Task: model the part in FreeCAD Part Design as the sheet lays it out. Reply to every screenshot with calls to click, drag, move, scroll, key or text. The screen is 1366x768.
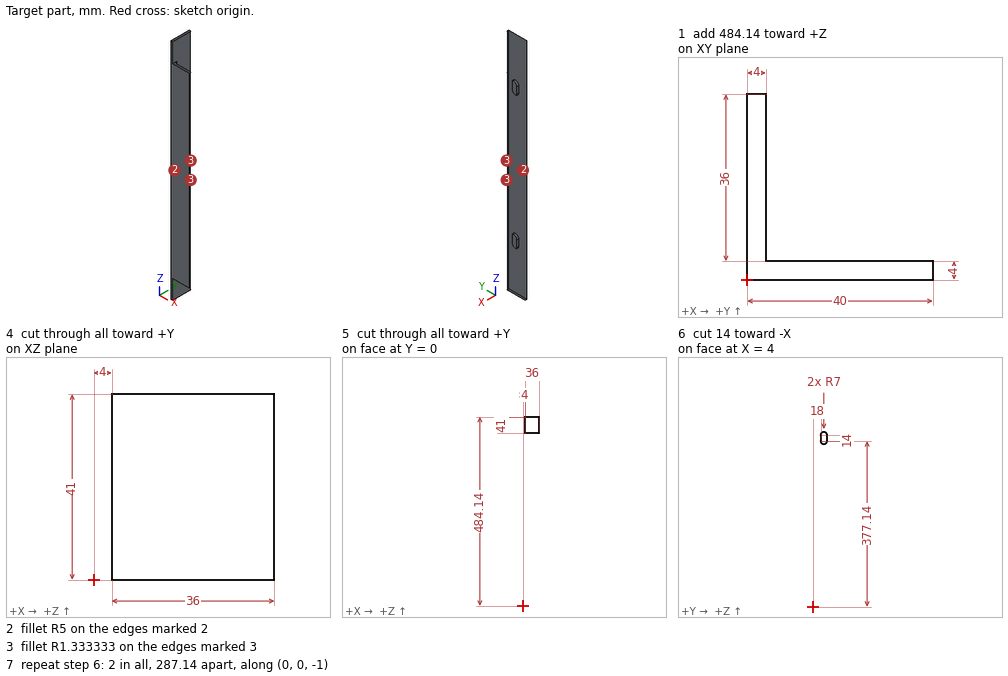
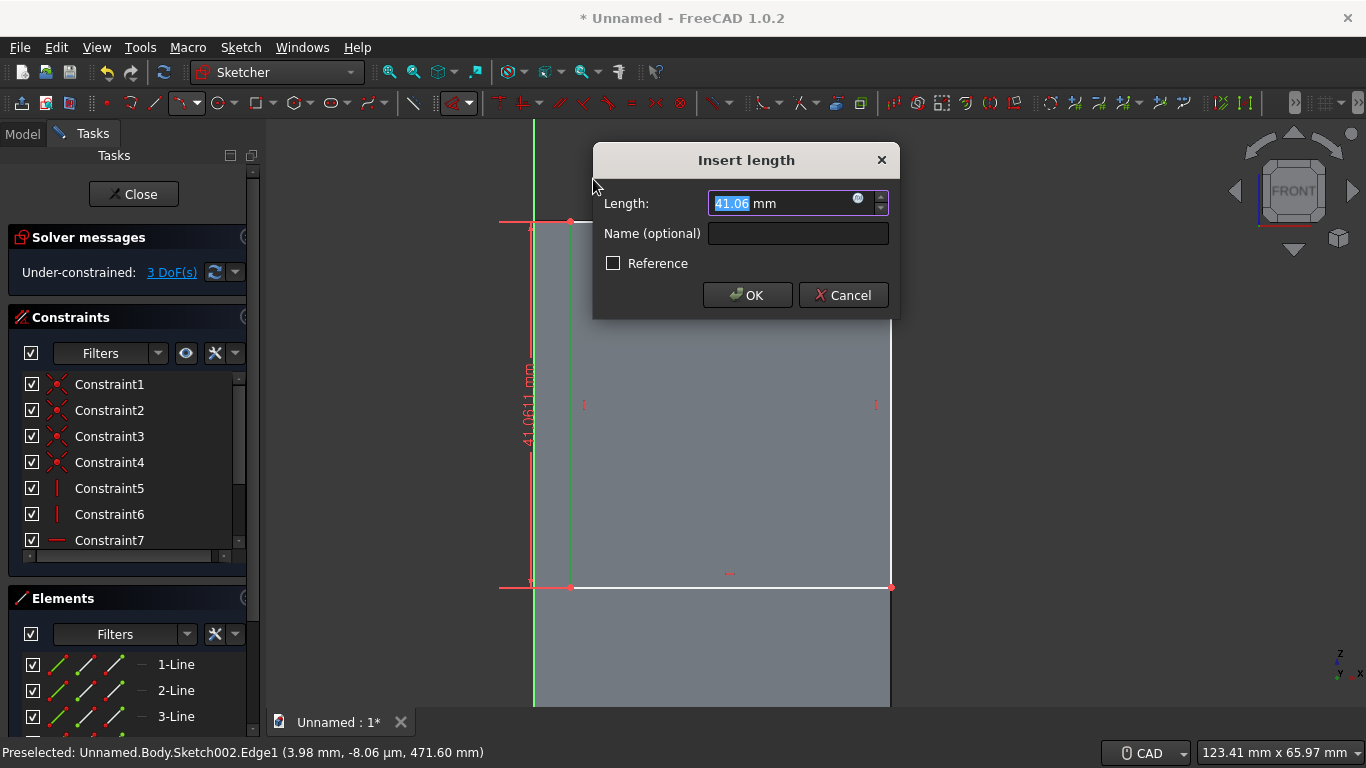
text(41)
key(Return)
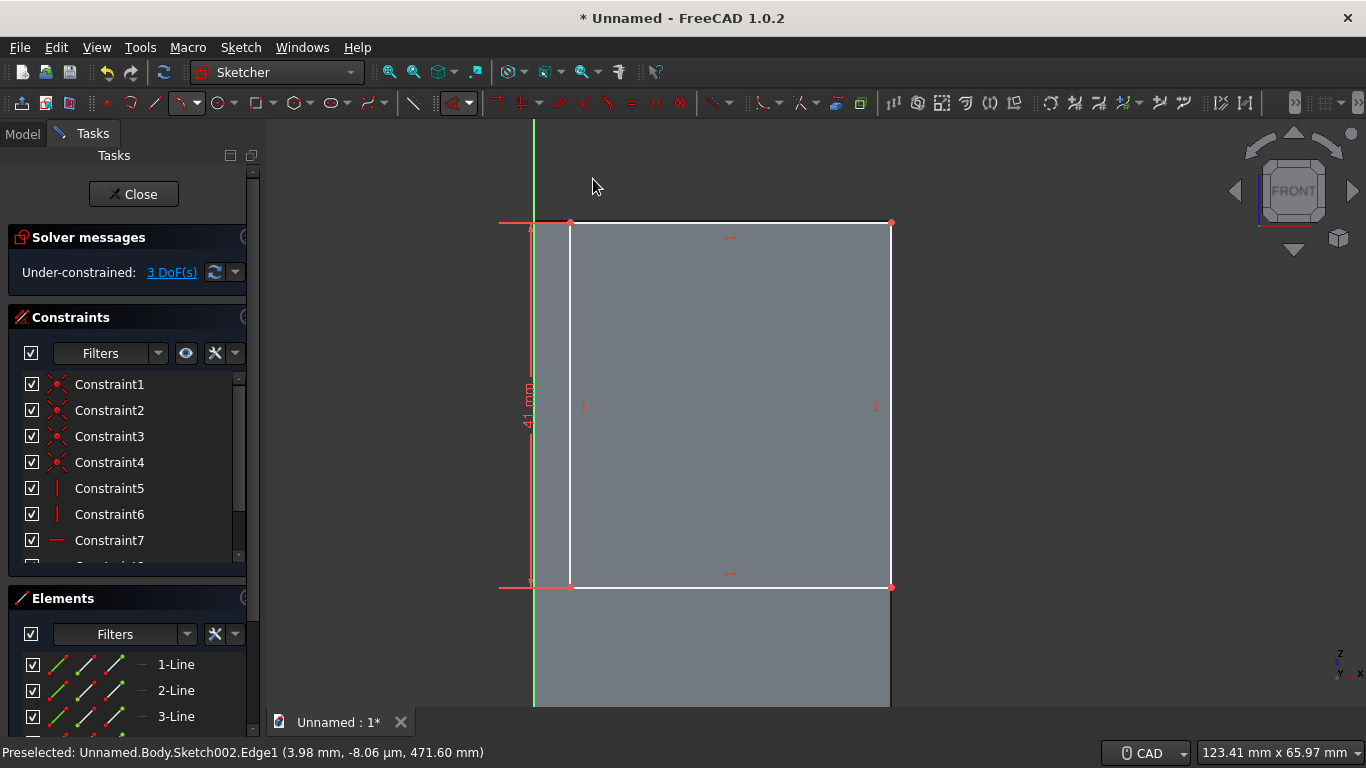
click(666, 588)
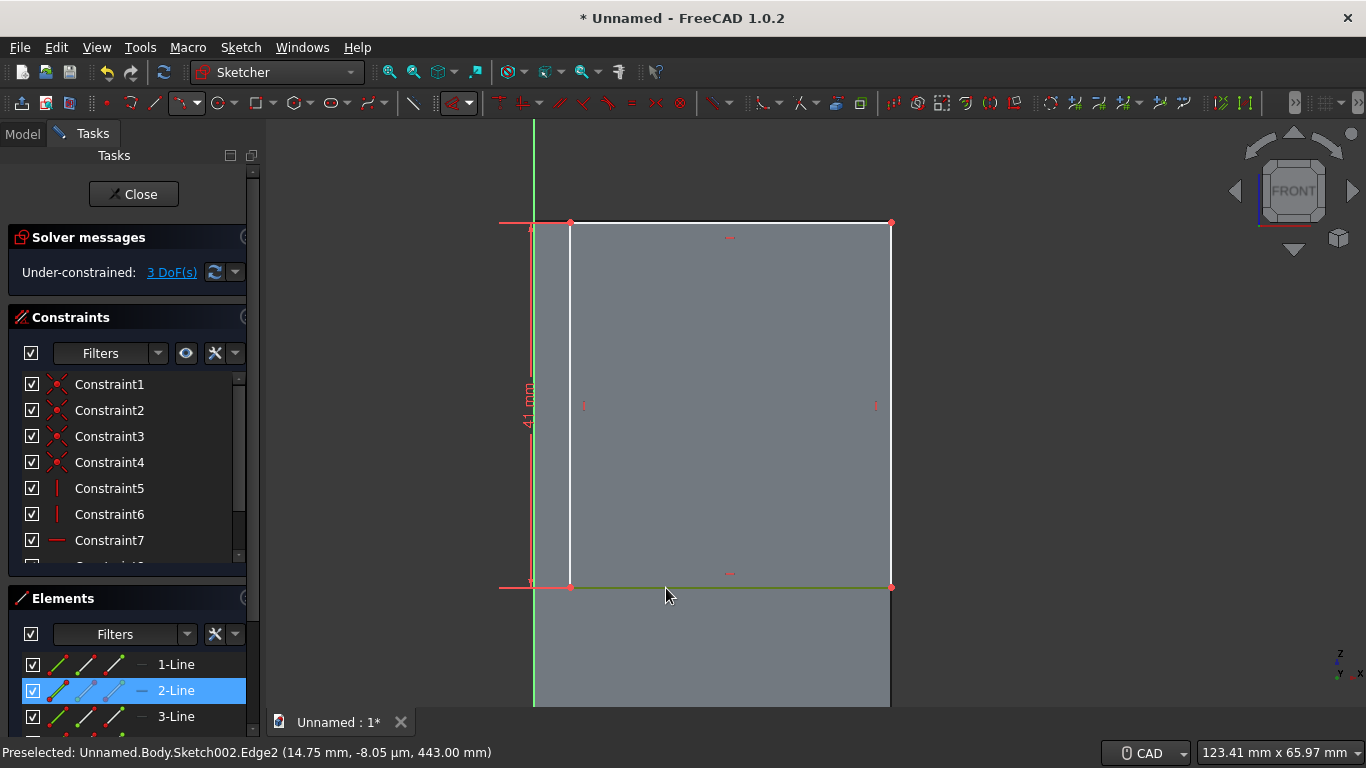
click(472, 104)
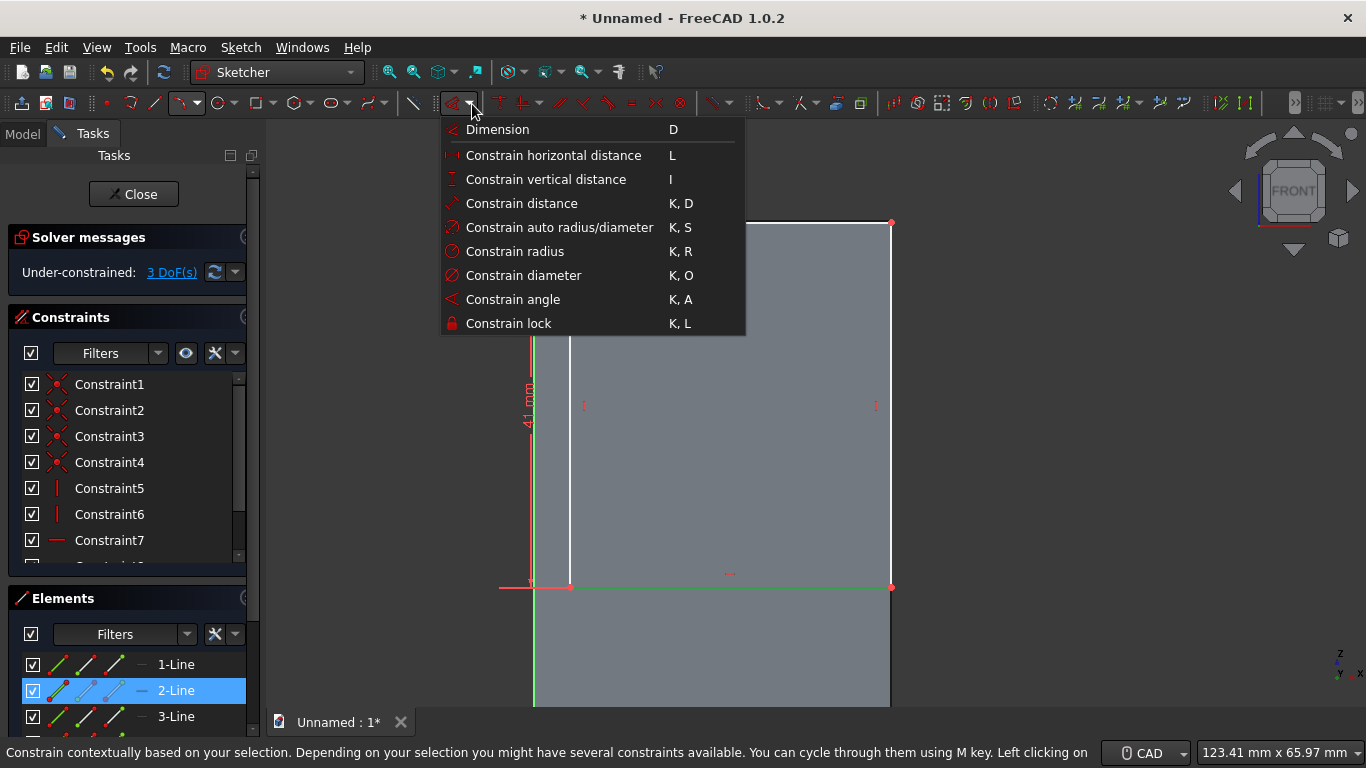
click(593, 155)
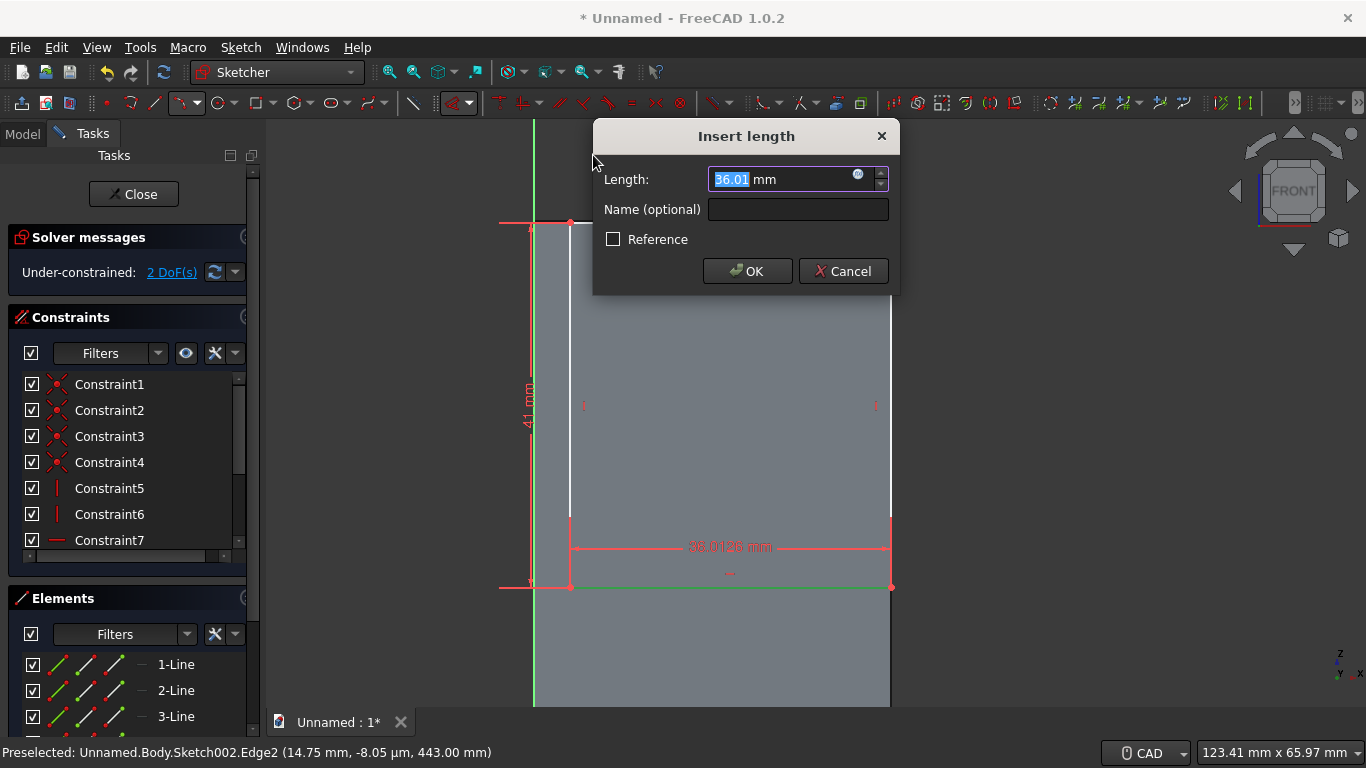
text(36)
key(Return)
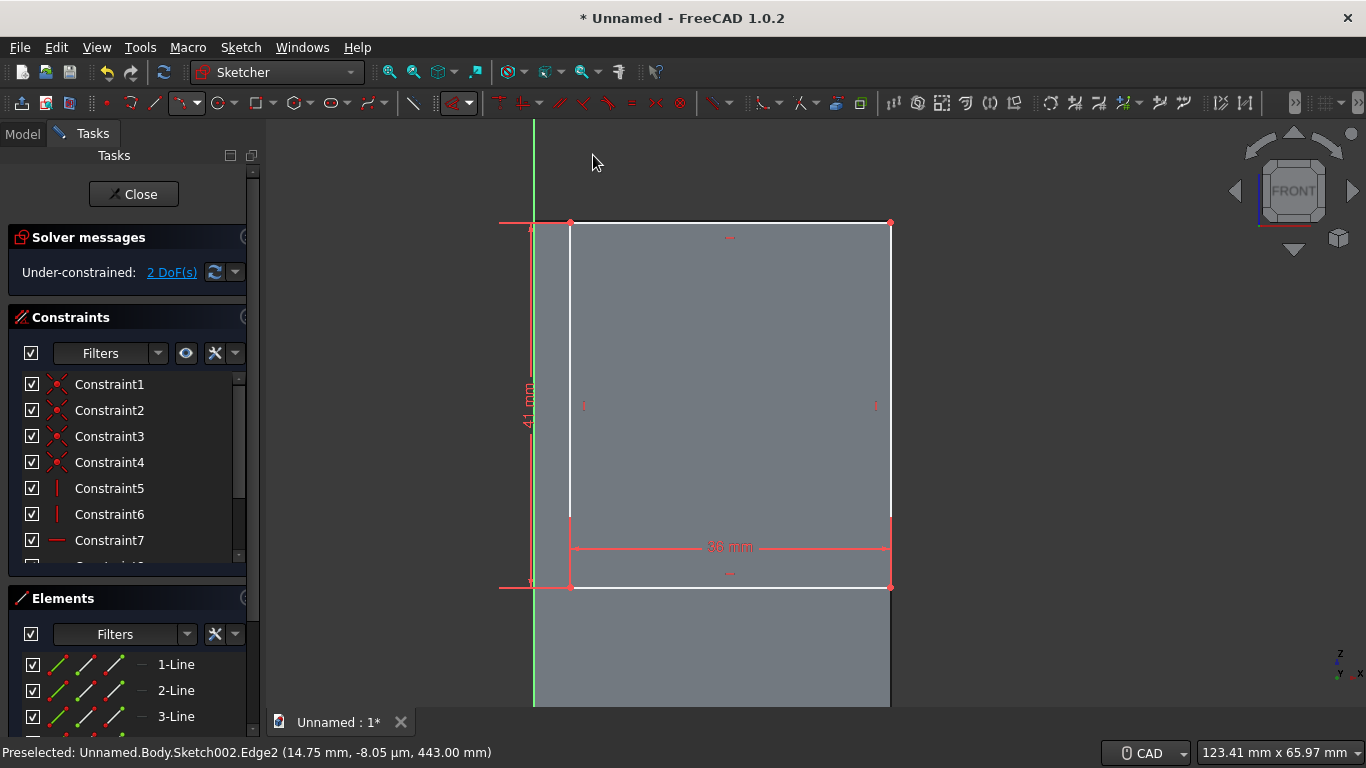
click(570, 223)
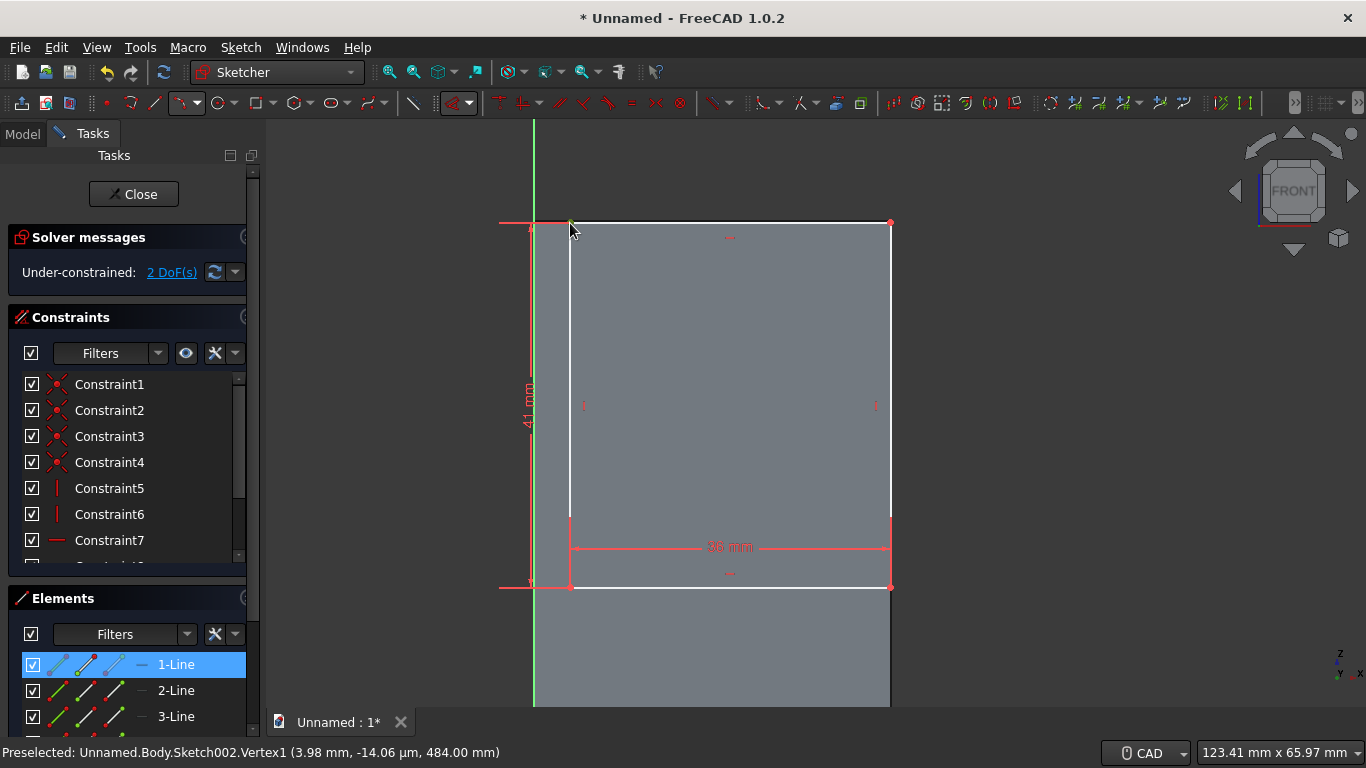
key(l)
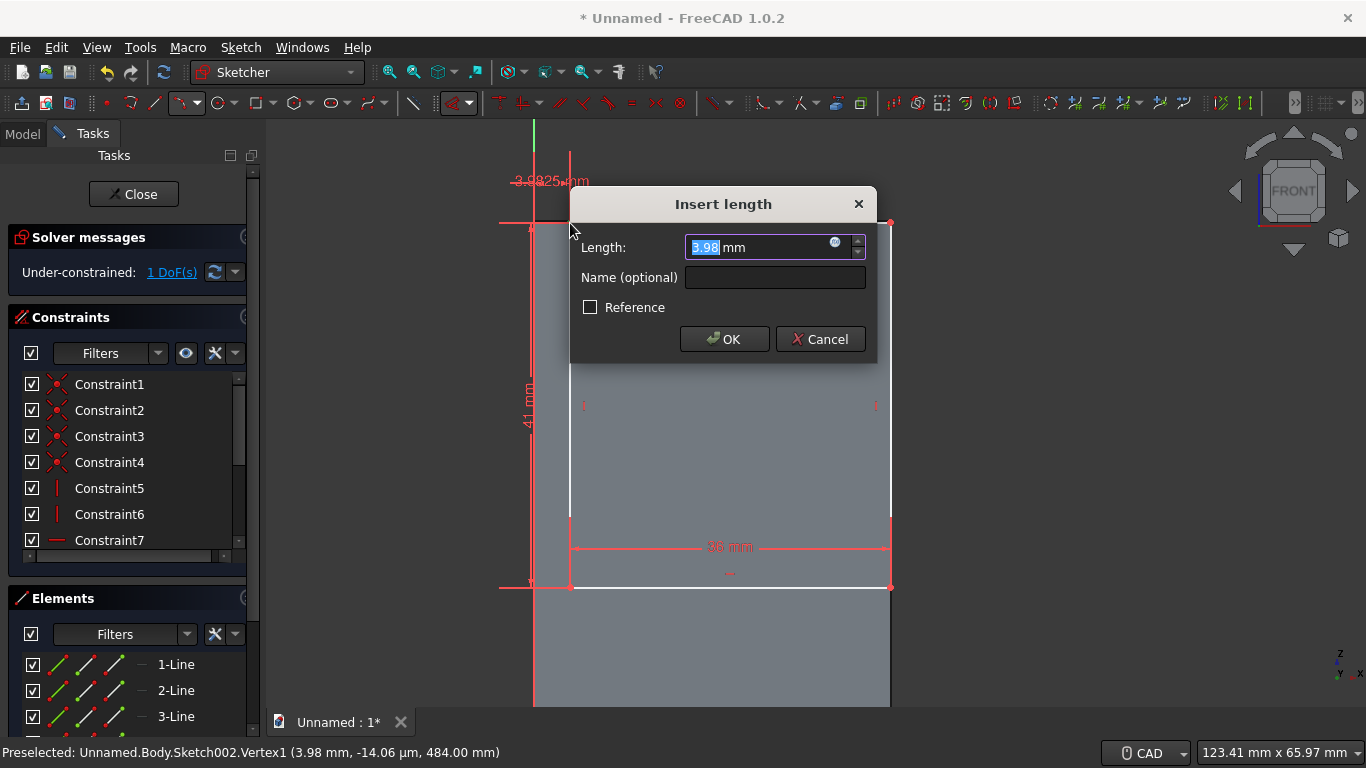
text(4)
key(Return)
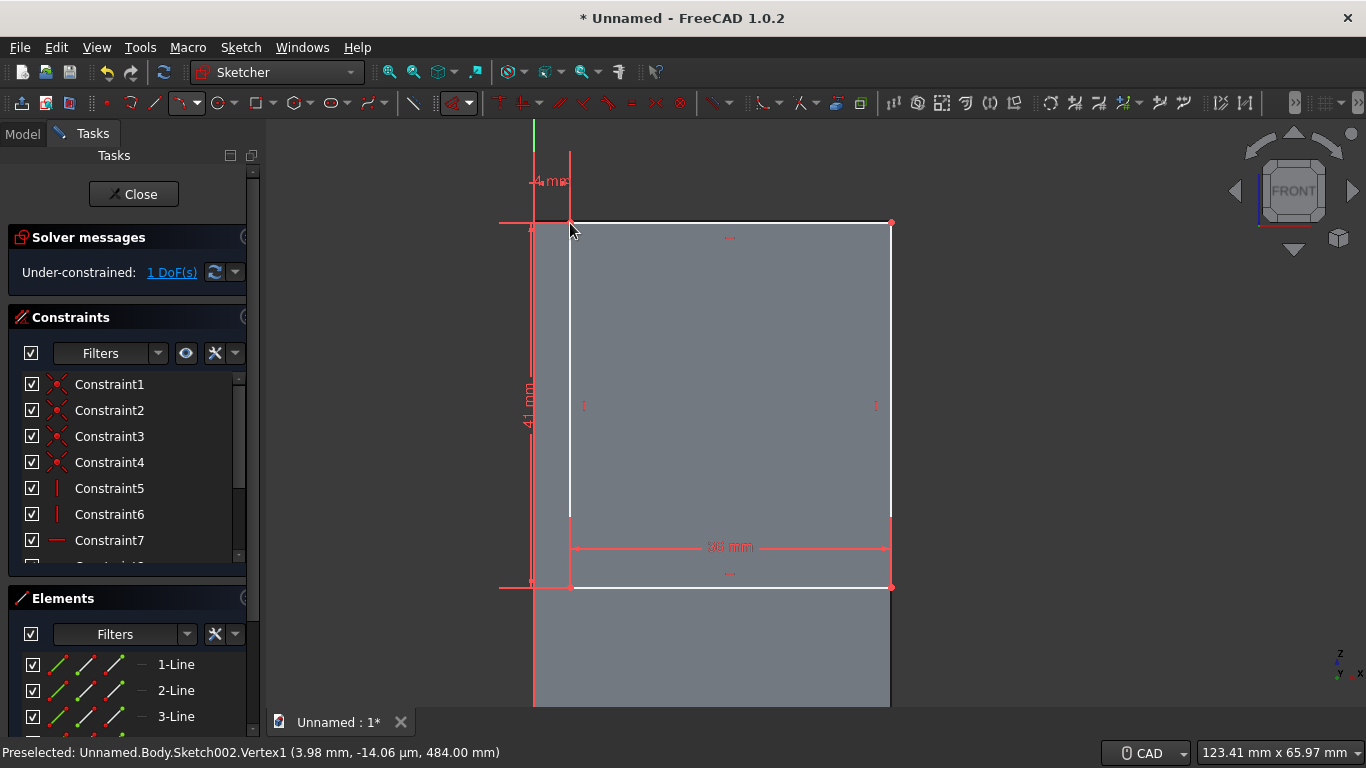
click(570, 223)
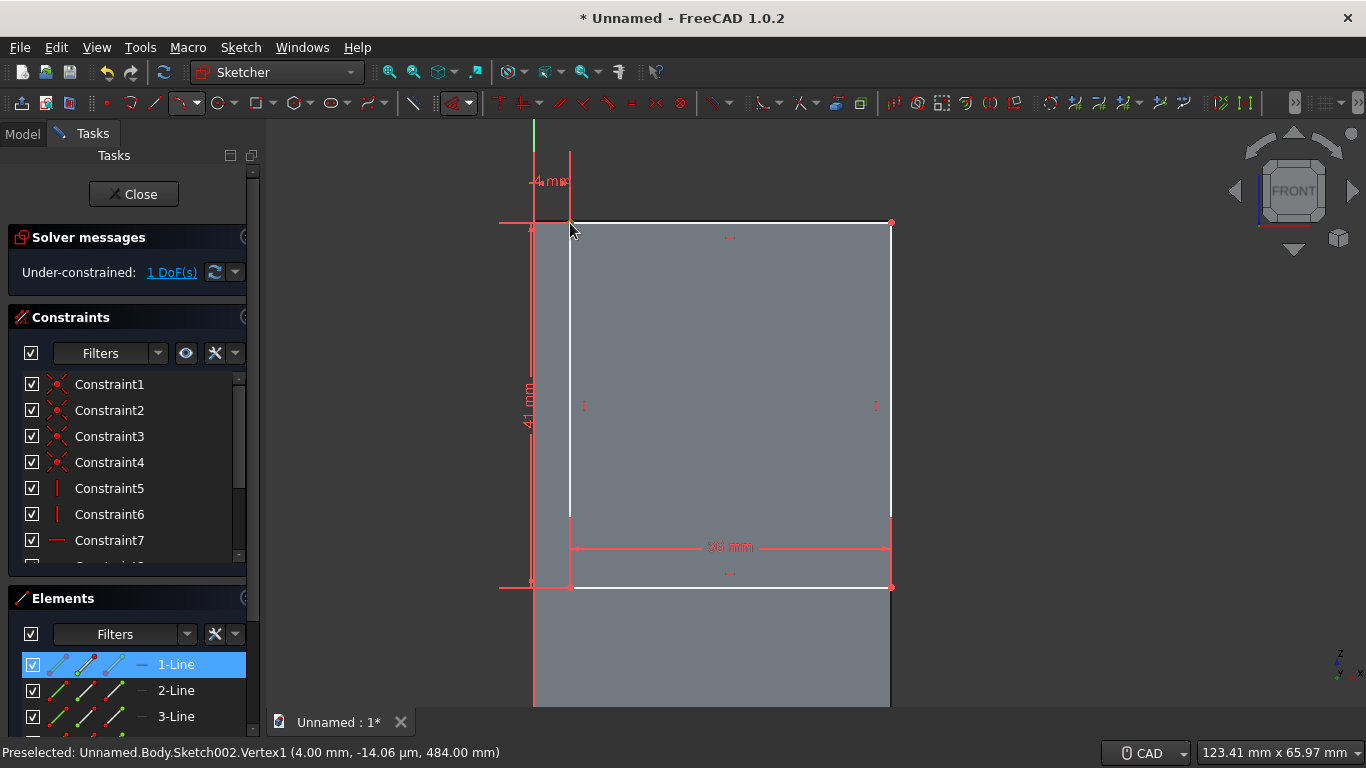
key(i)